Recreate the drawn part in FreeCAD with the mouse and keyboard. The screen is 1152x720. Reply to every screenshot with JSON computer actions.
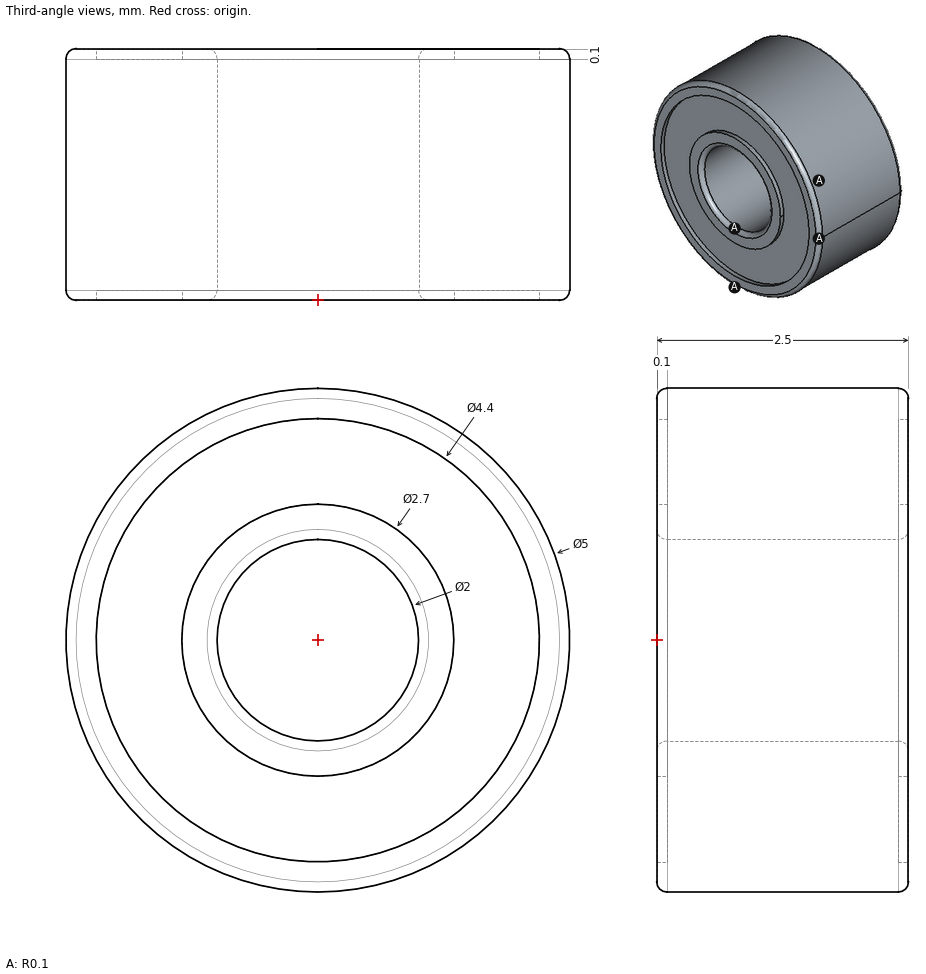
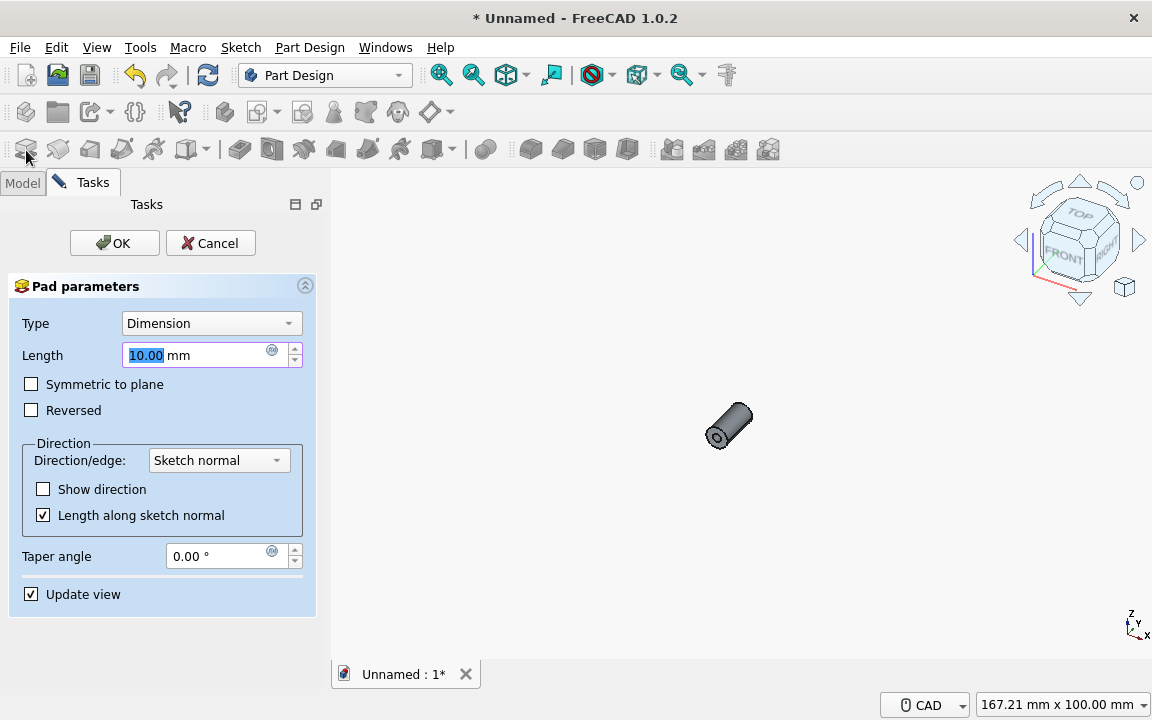
{"action": "type", "text": "2.5"}
{"action": "key", "text": "Tab"}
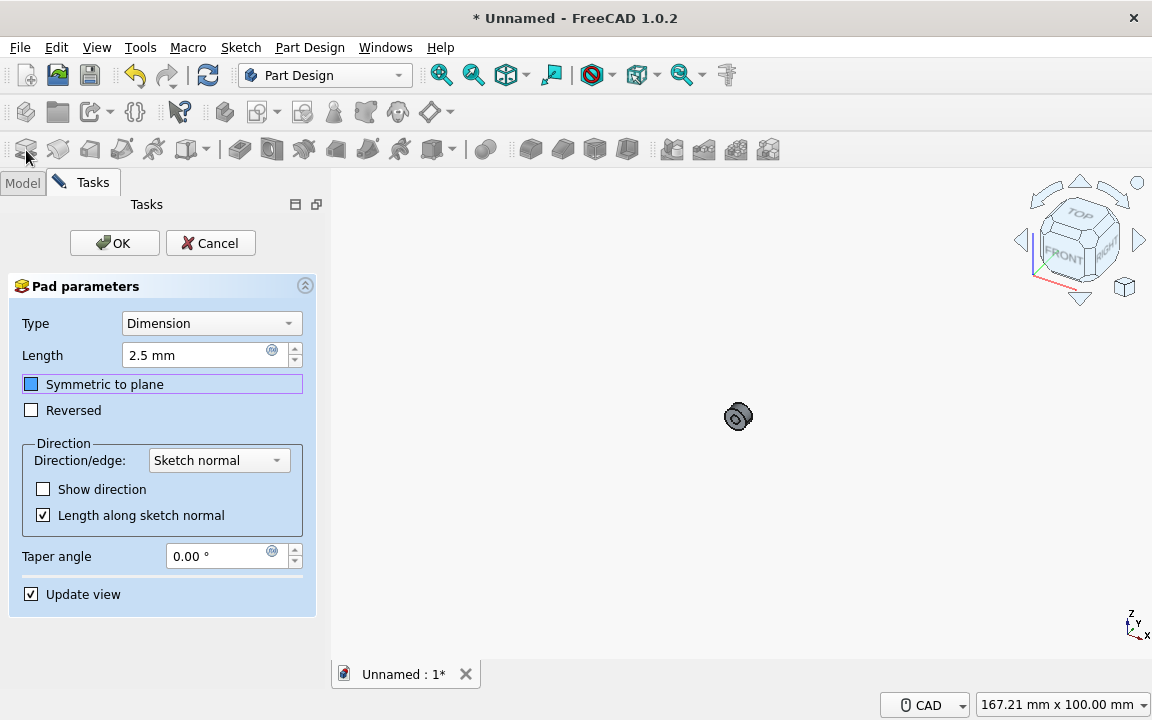
{"action": "left_click", "coordinate": [30, 410]}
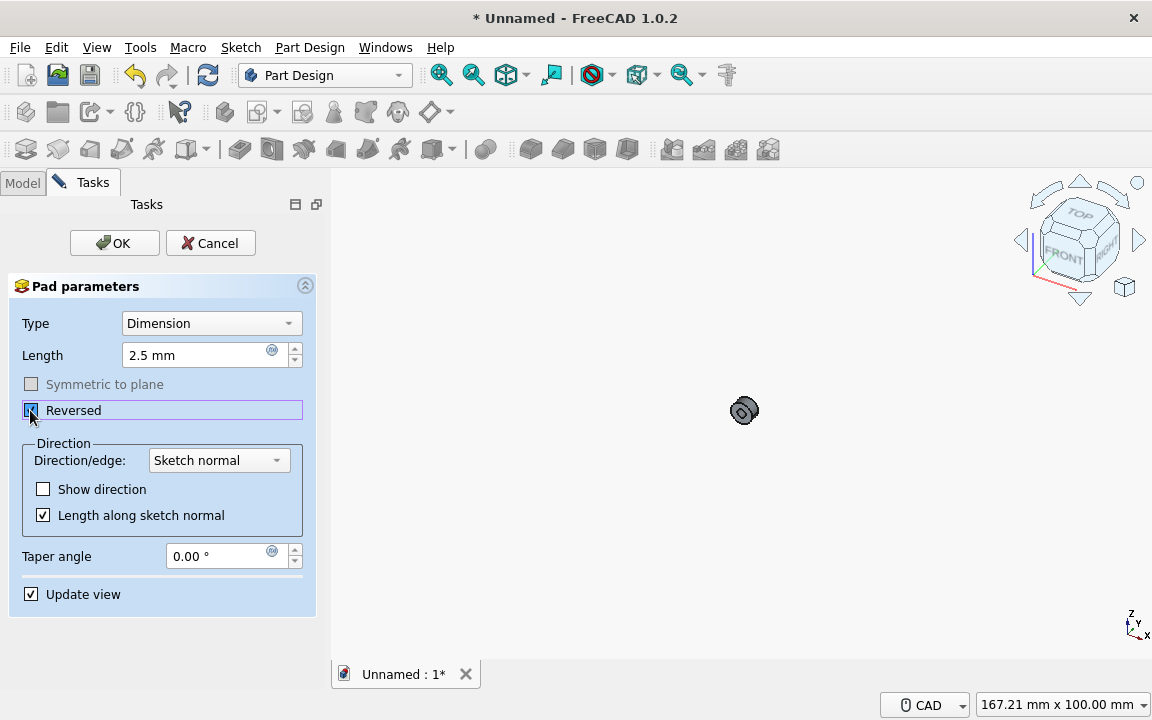
{"action": "left_click", "coordinate": [115, 243]}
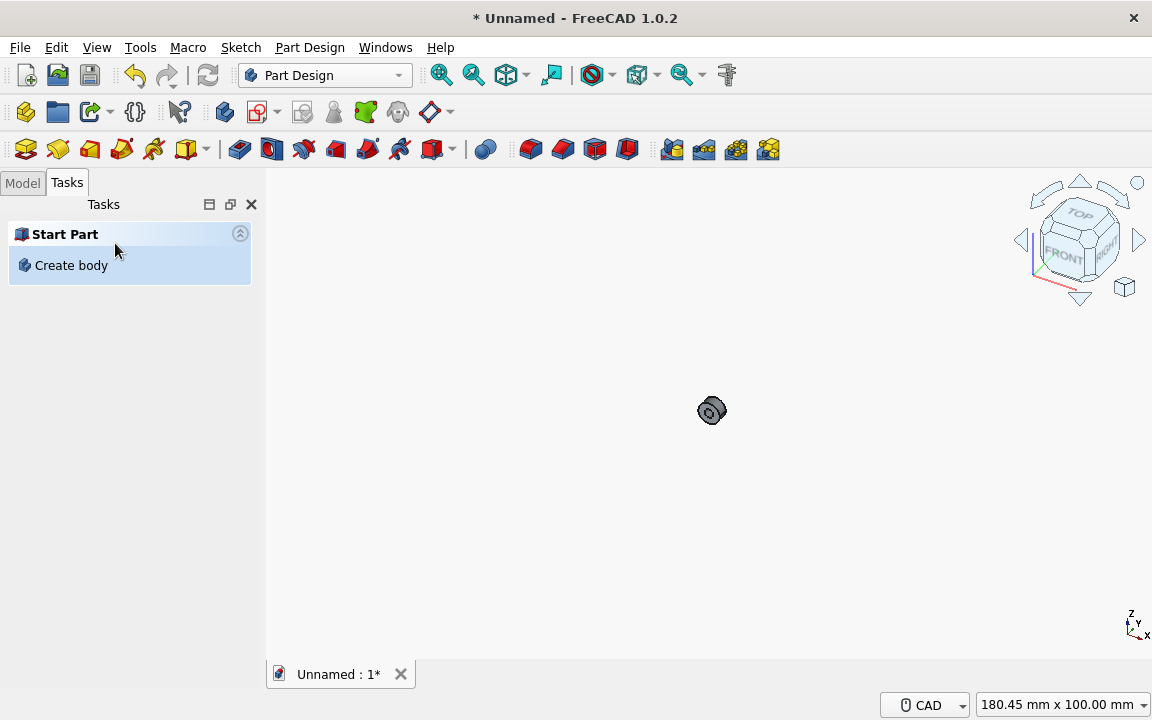
{"action": "left_click", "coordinate": [442, 76]}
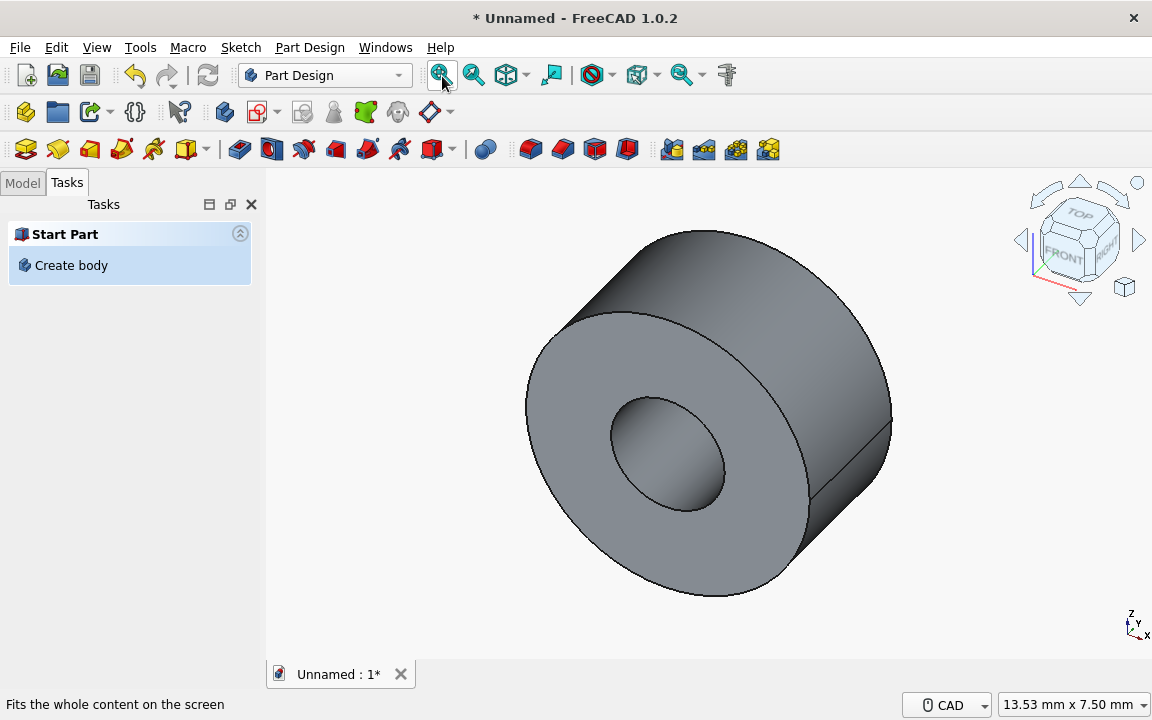
{"action": "key", "text": "4"}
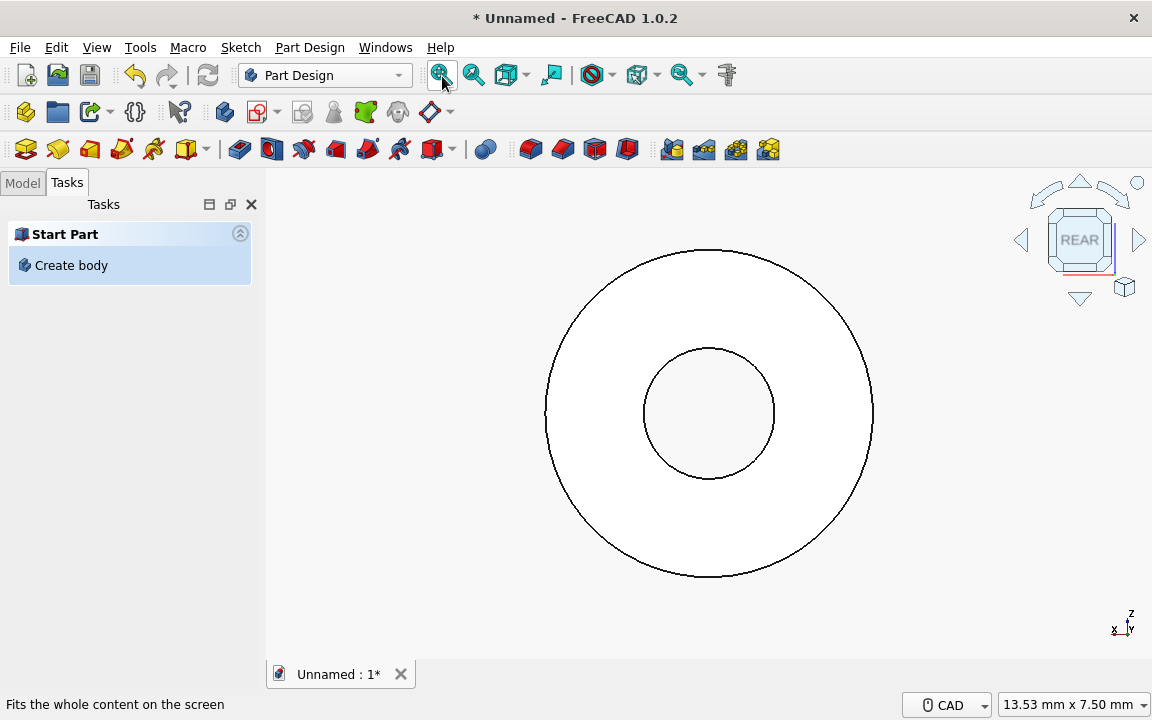
{"action": "left_click", "coordinate": [803, 366]}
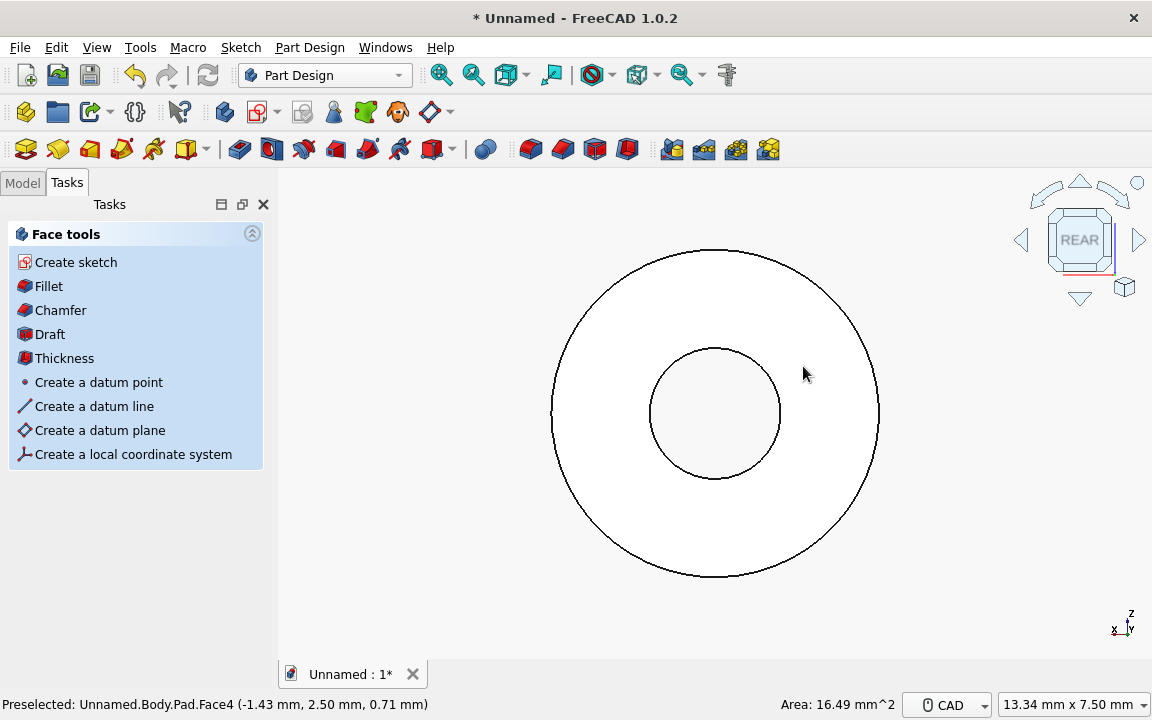
{"action": "left_click", "coordinate": [258, 112]}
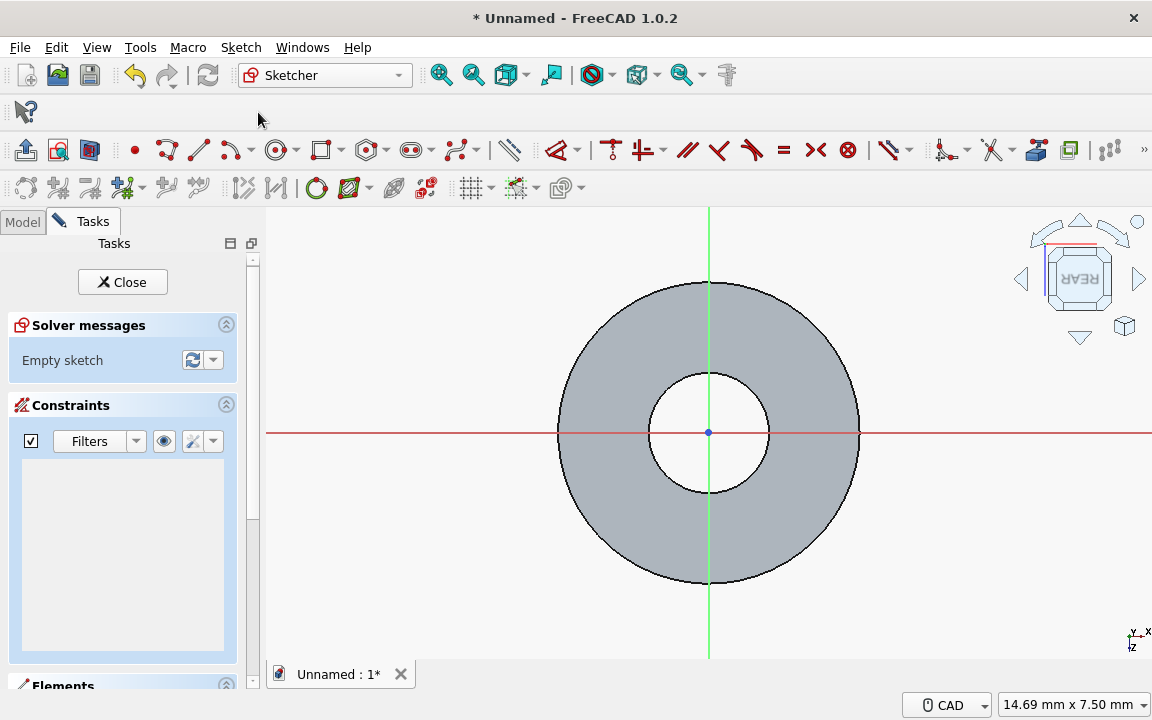
{"action": "left_click", "coordinate": [276, 150]}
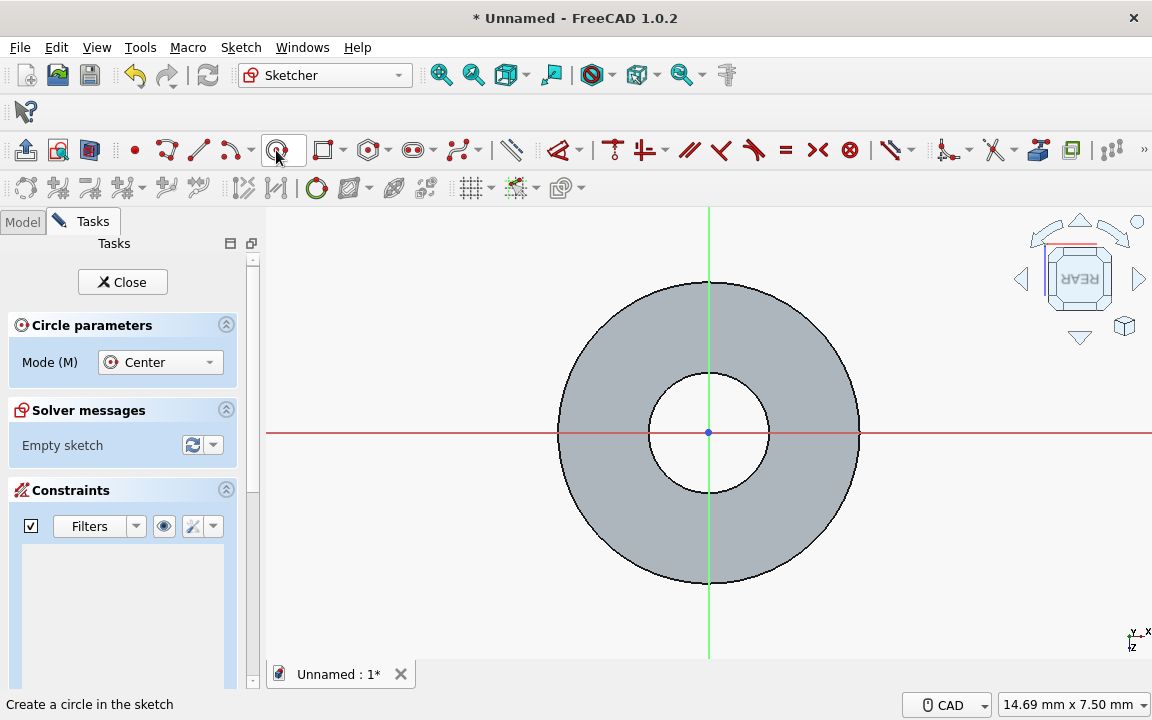
{"action": "left_click", "coordinate": [709, 433]}
{"action": "mouse_move", "coordinate": [803, 339]}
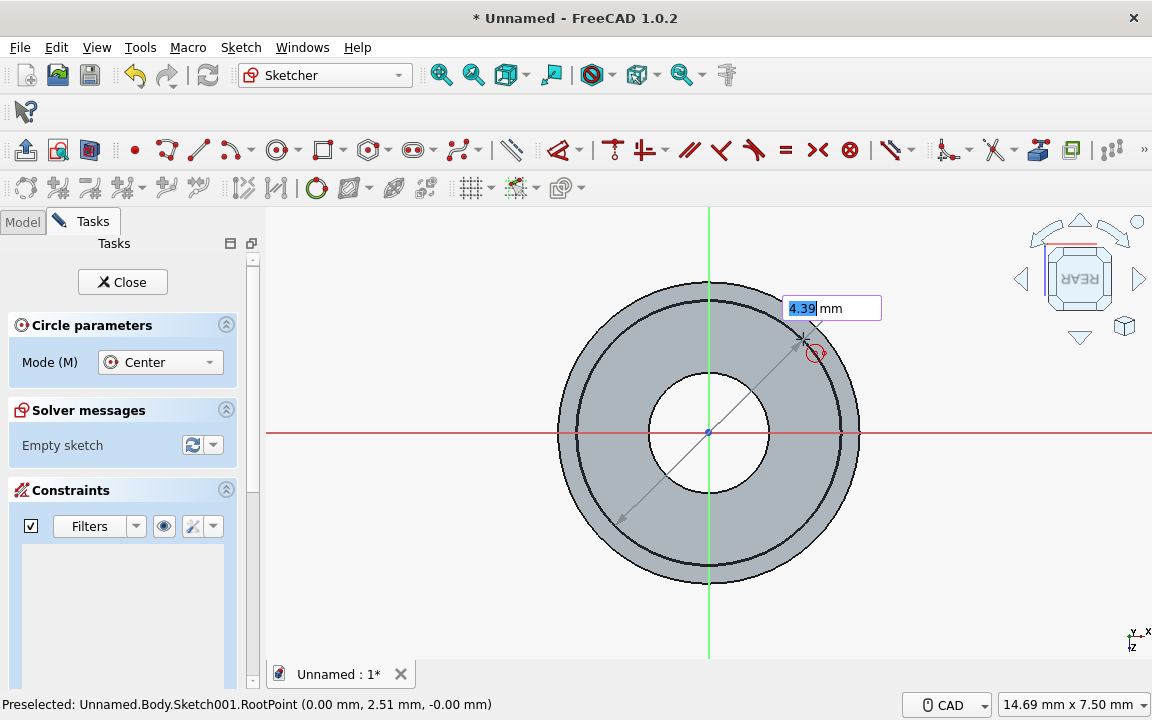
{"action": "type", "text": "4.4"}
{"action": "key", "text": "Return"}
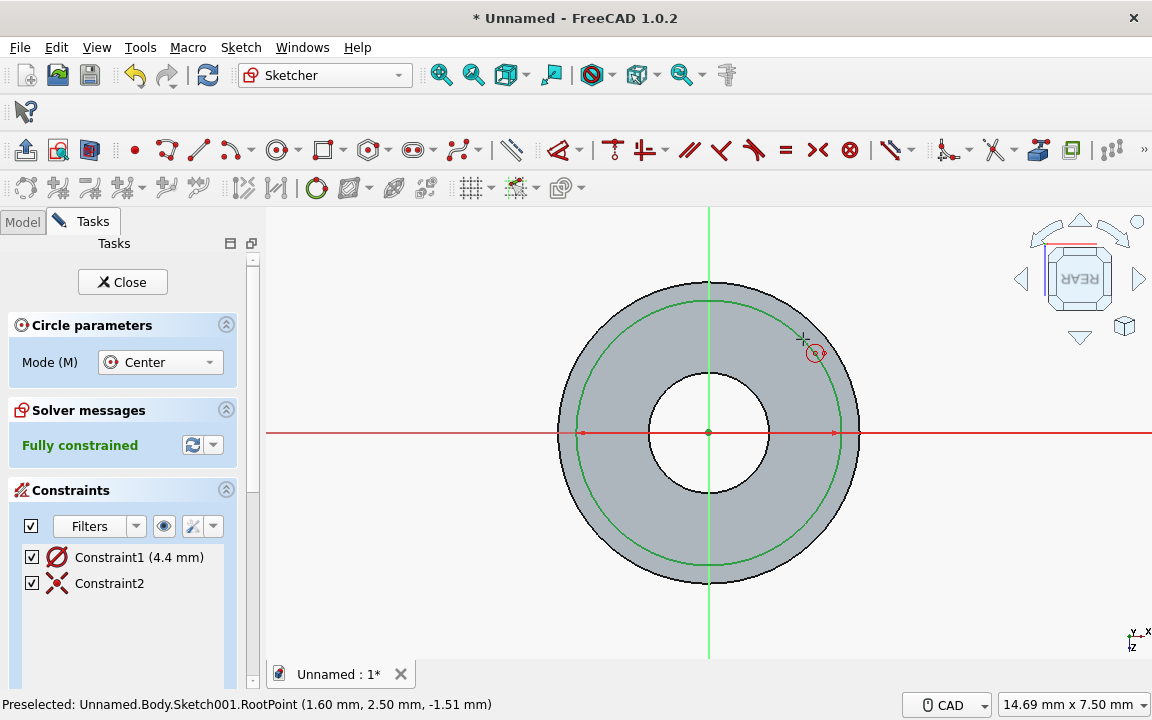
{"action": "left_click", "coordinate": [709, 433]}
{"action": "mouse_move", "coordinate": [766, 375]}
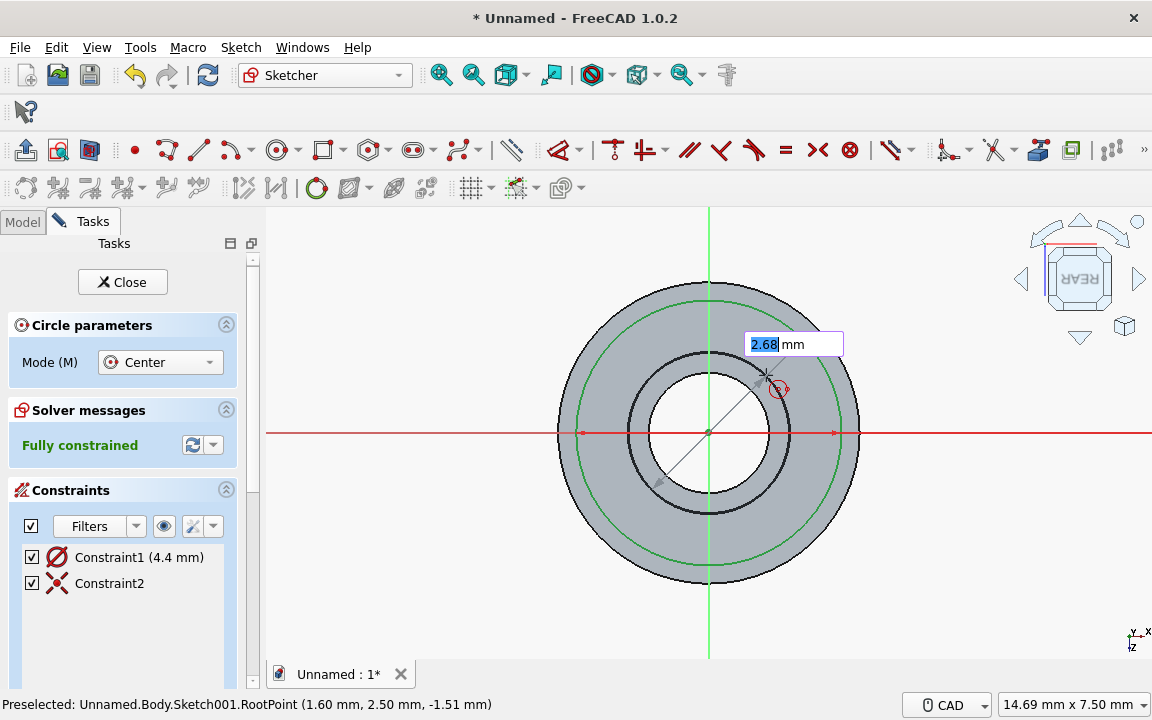
{"action": "type", "text": "2.7"}
{"action": "key", "text": "Return"}
{"action": "key", "text": "Escape"}